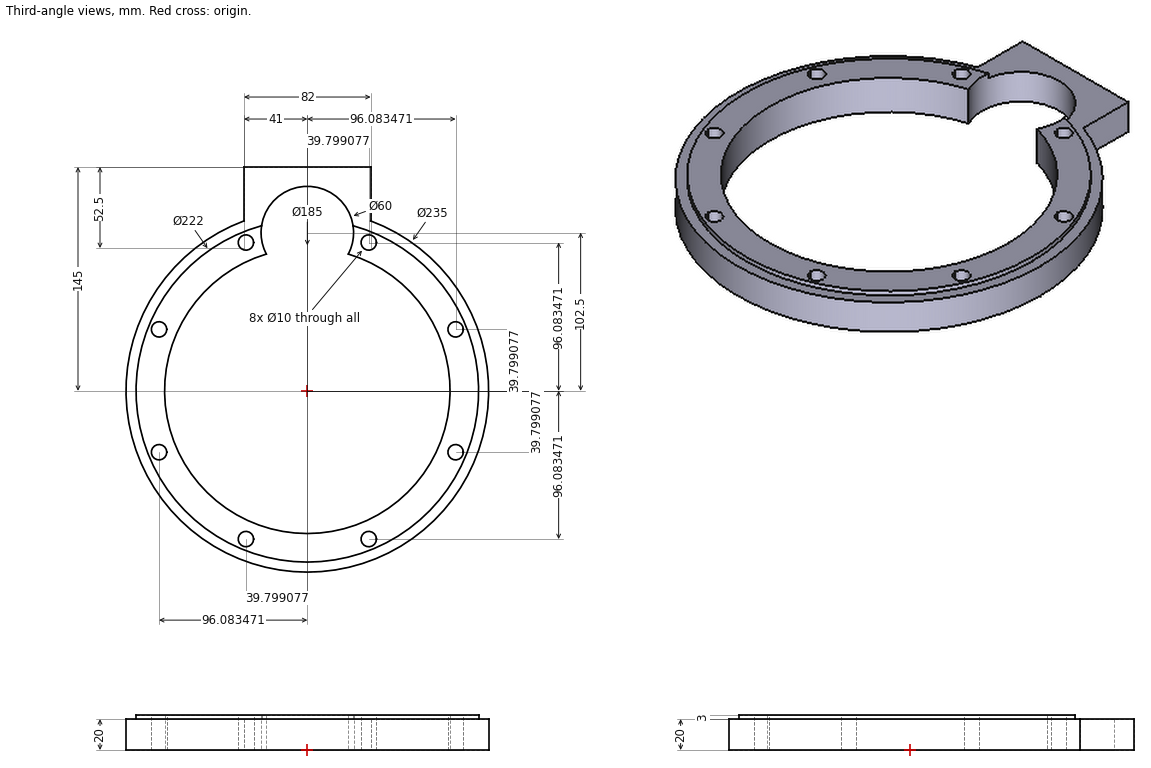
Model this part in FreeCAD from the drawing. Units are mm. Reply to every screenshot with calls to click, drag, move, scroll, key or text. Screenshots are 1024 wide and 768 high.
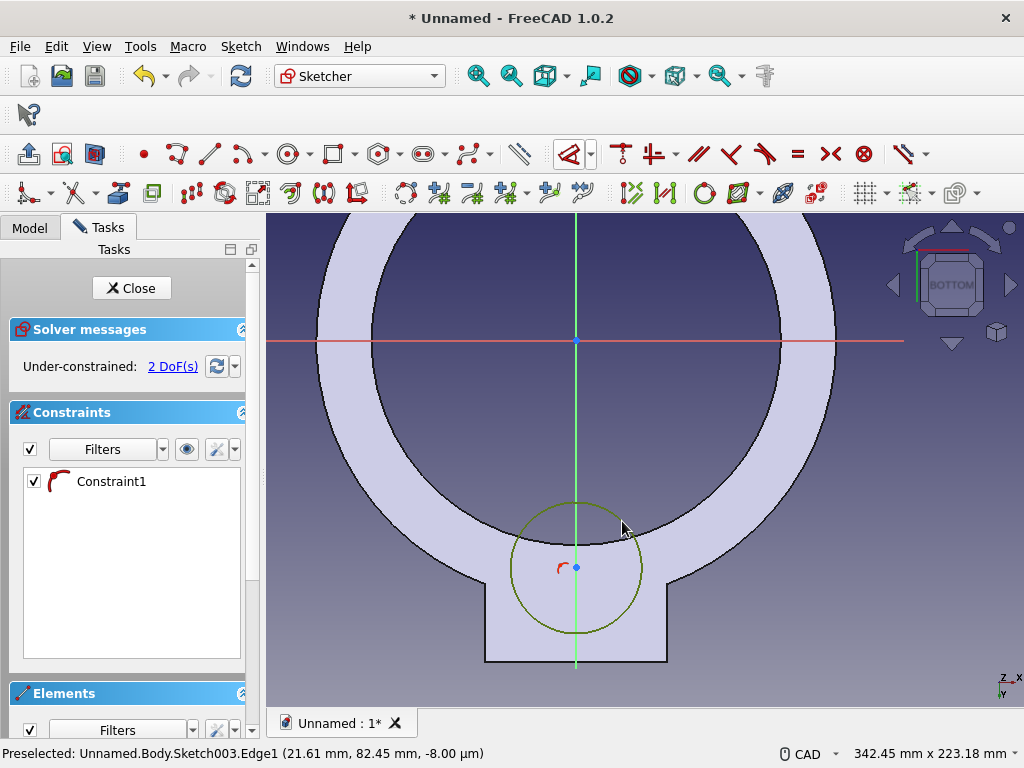
key(k)
key(o)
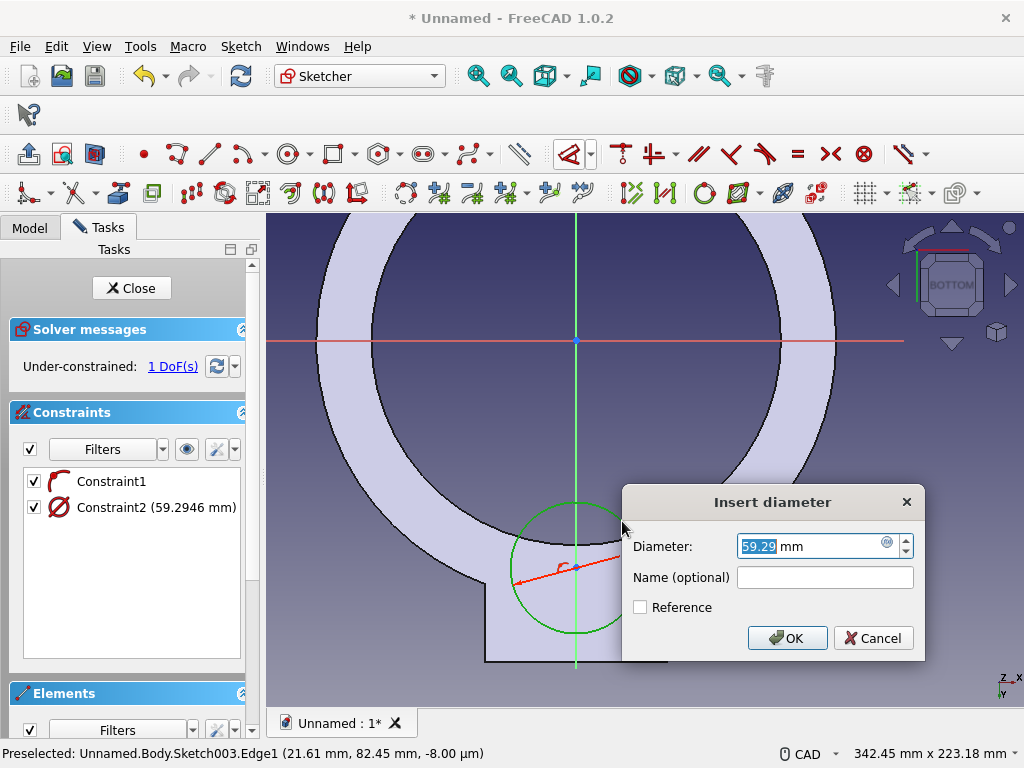
text(60)
key(Return)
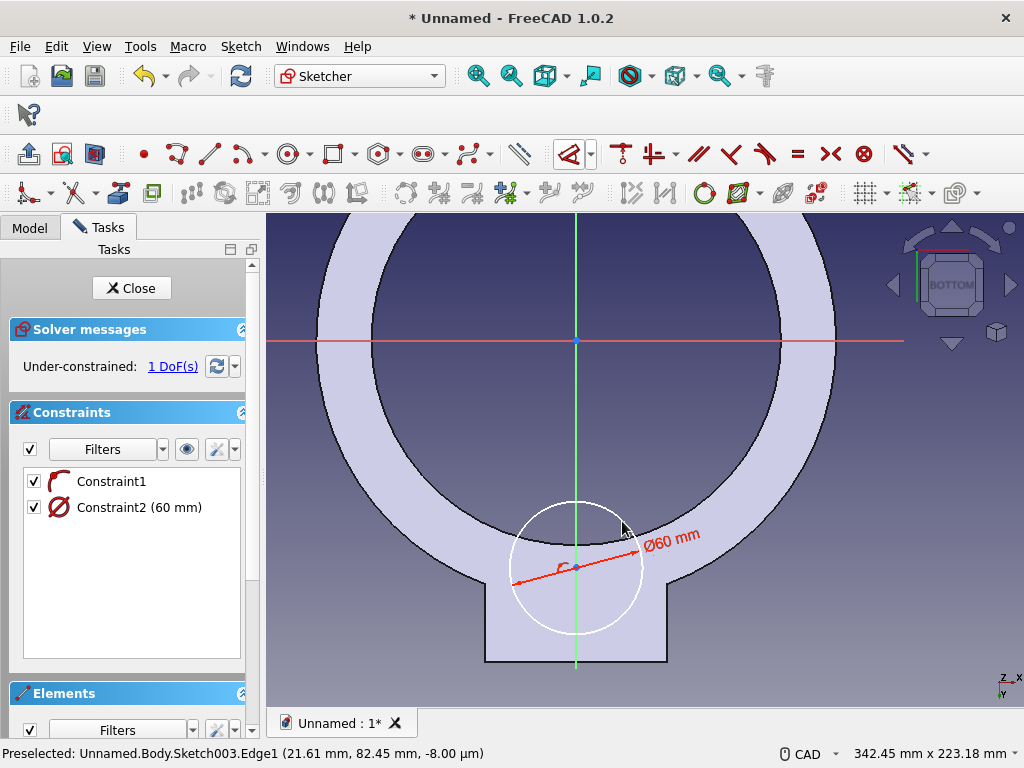
click(576, 568)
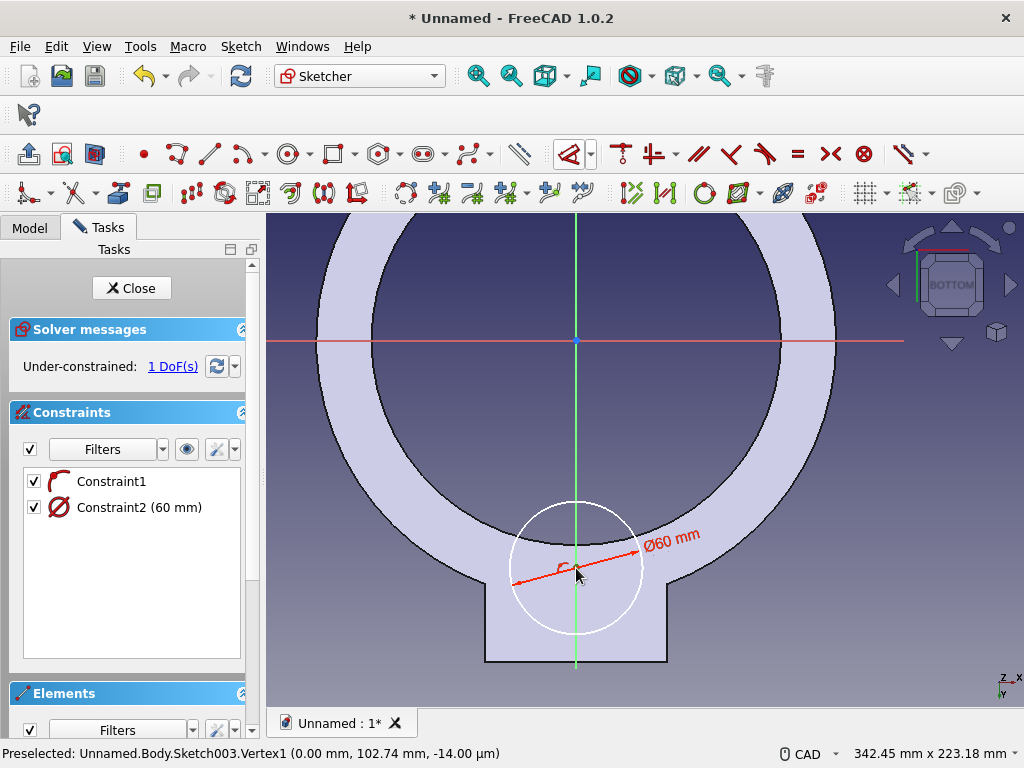
key(i)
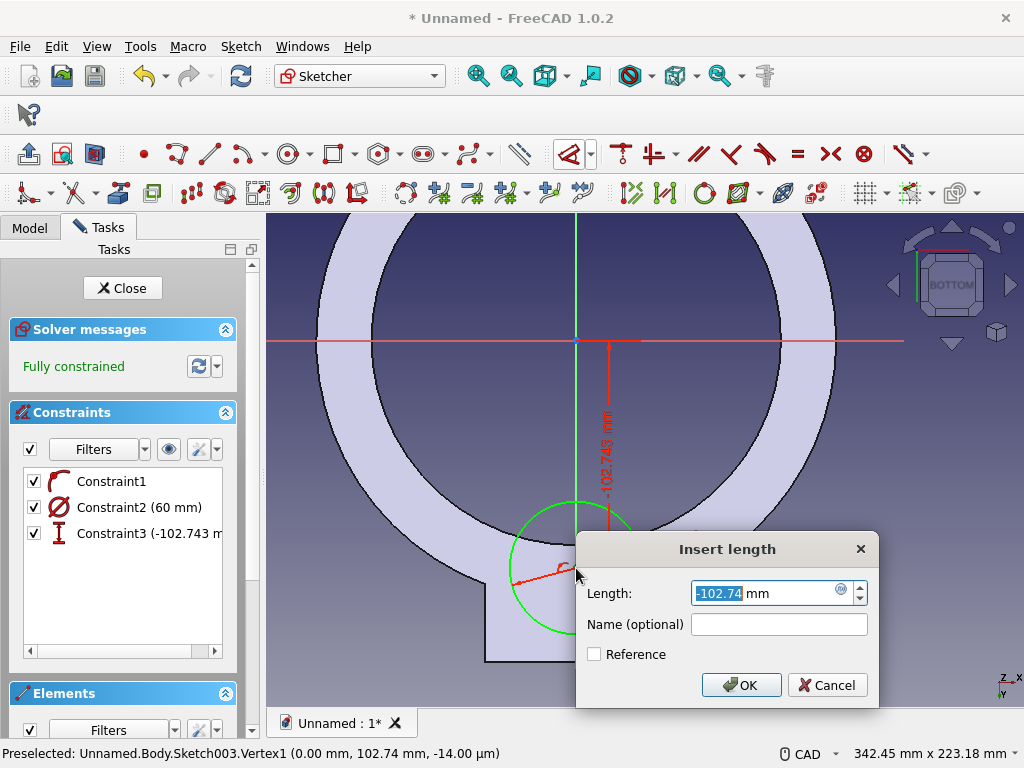
text(-102.5)
key(Return)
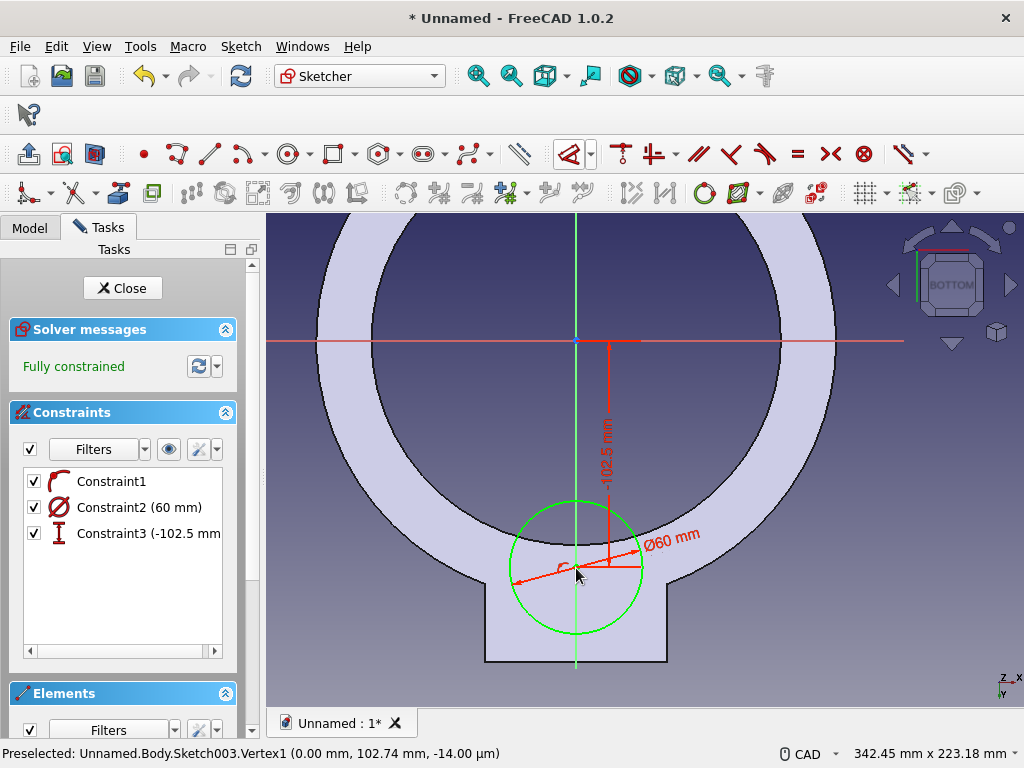
click(123, 288)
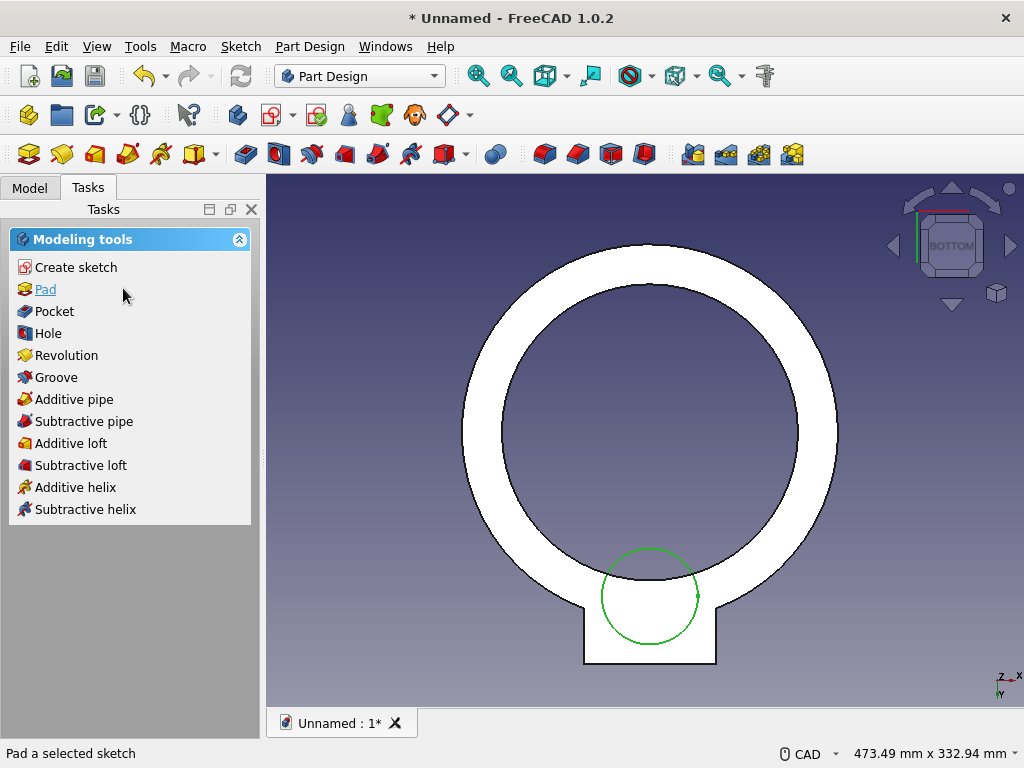
click(246, 154)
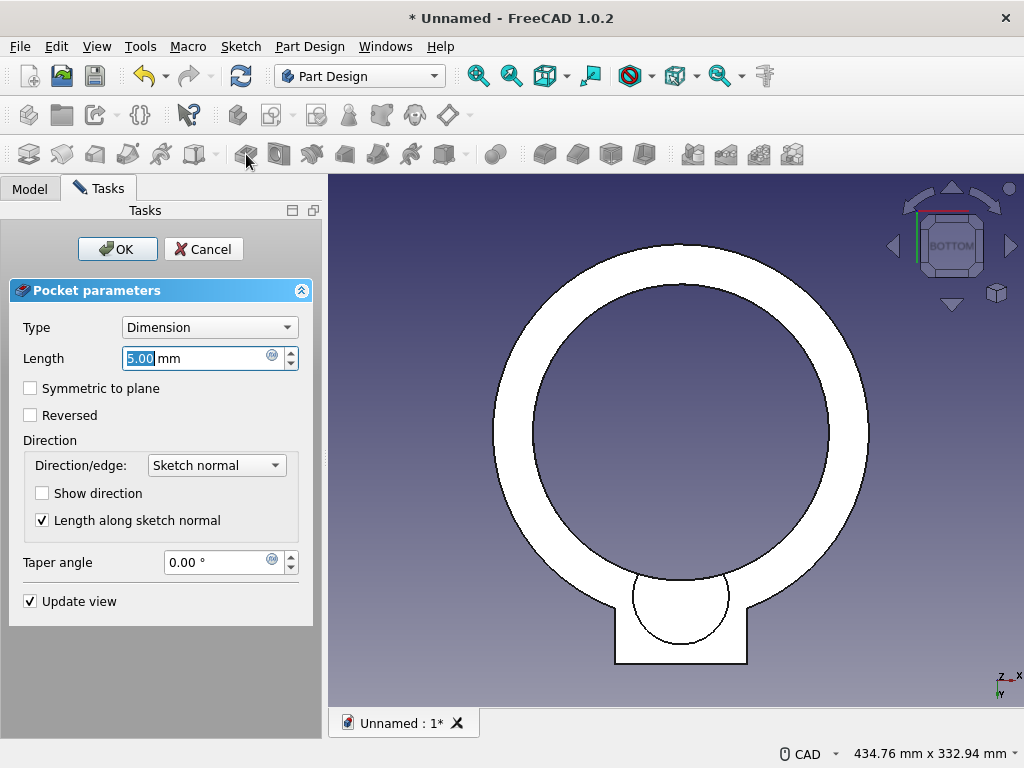
click(210, 328)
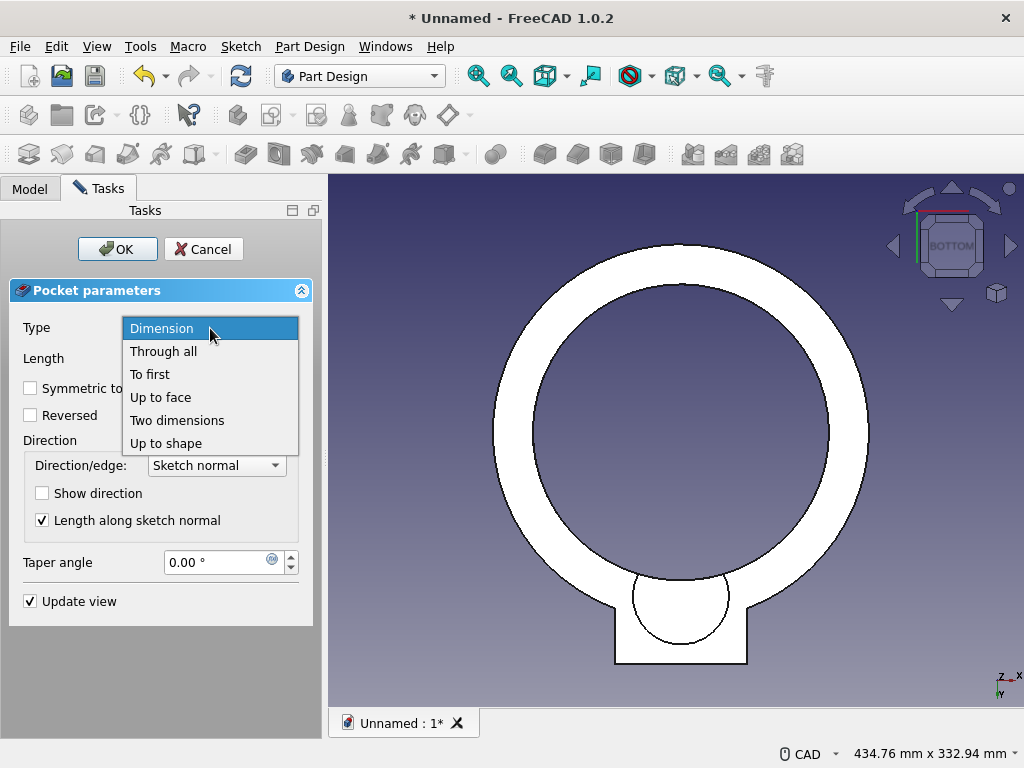
click(208, 352)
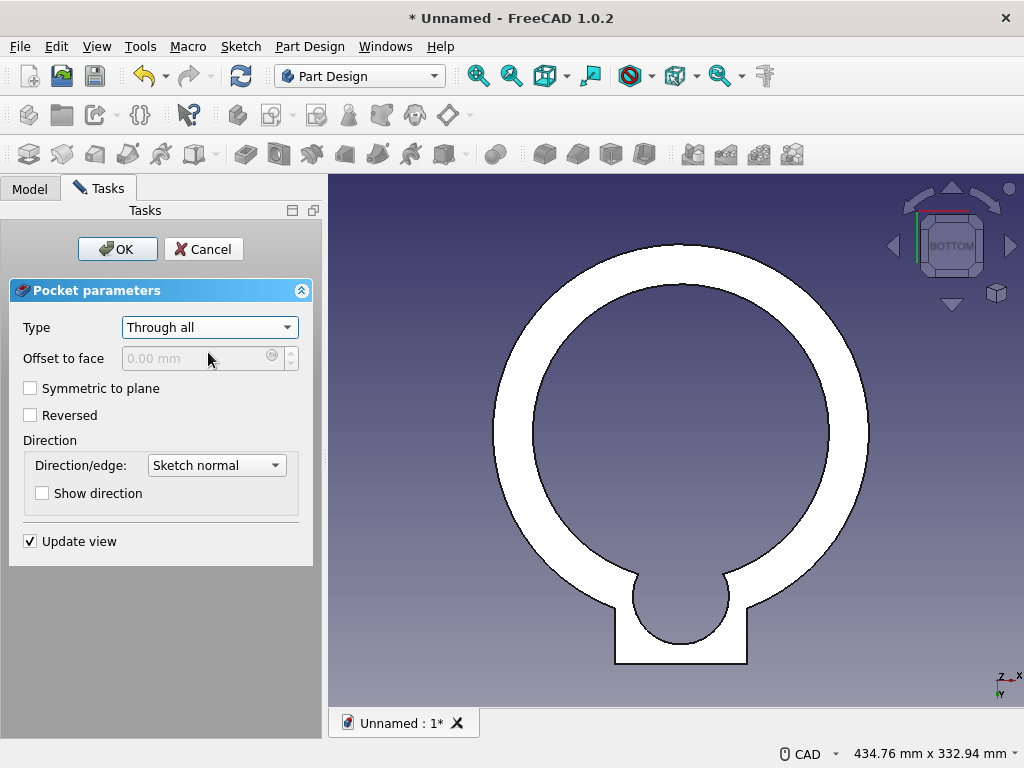
click(118, 249)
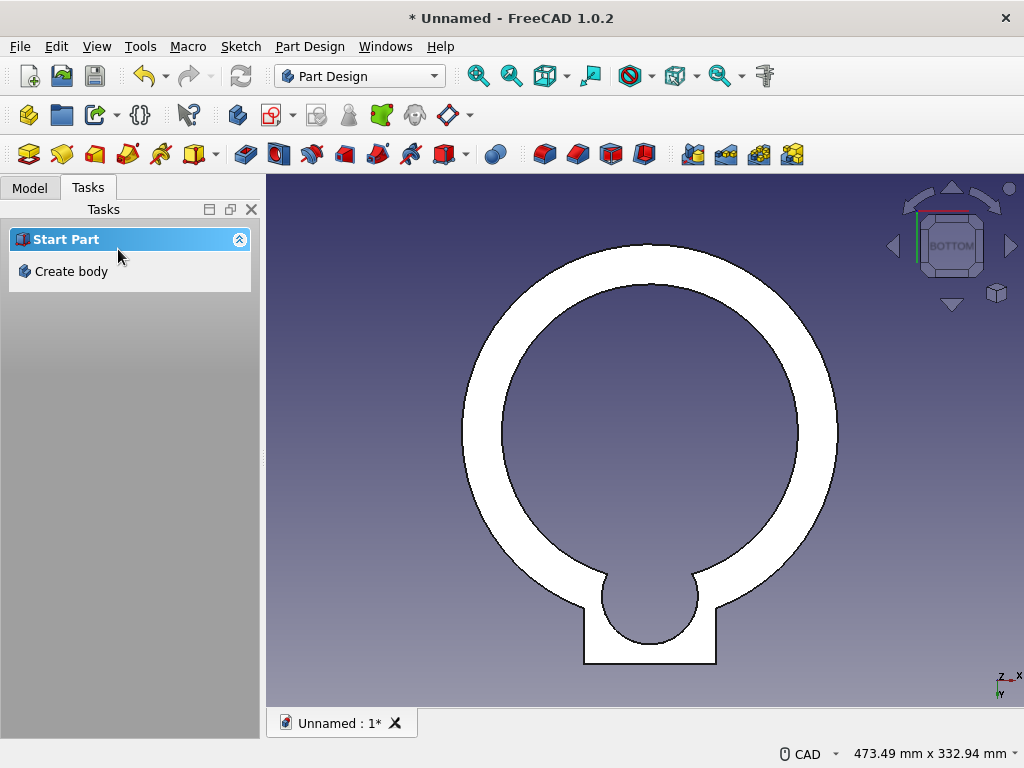
click(704, 273)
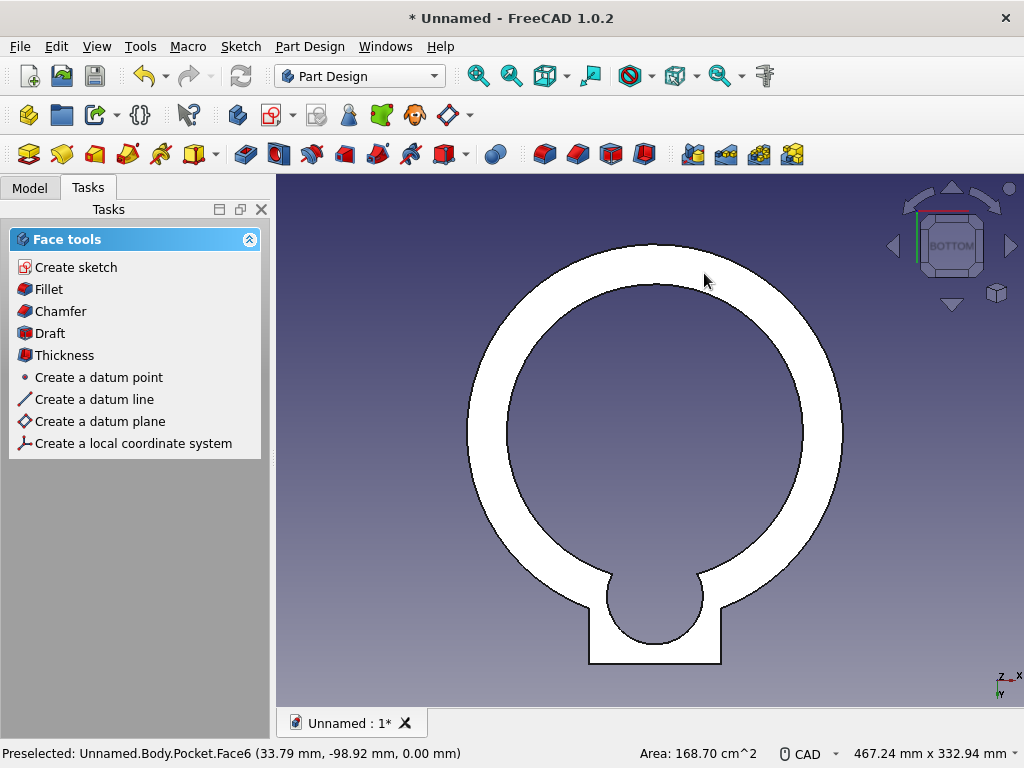
click(270, 116)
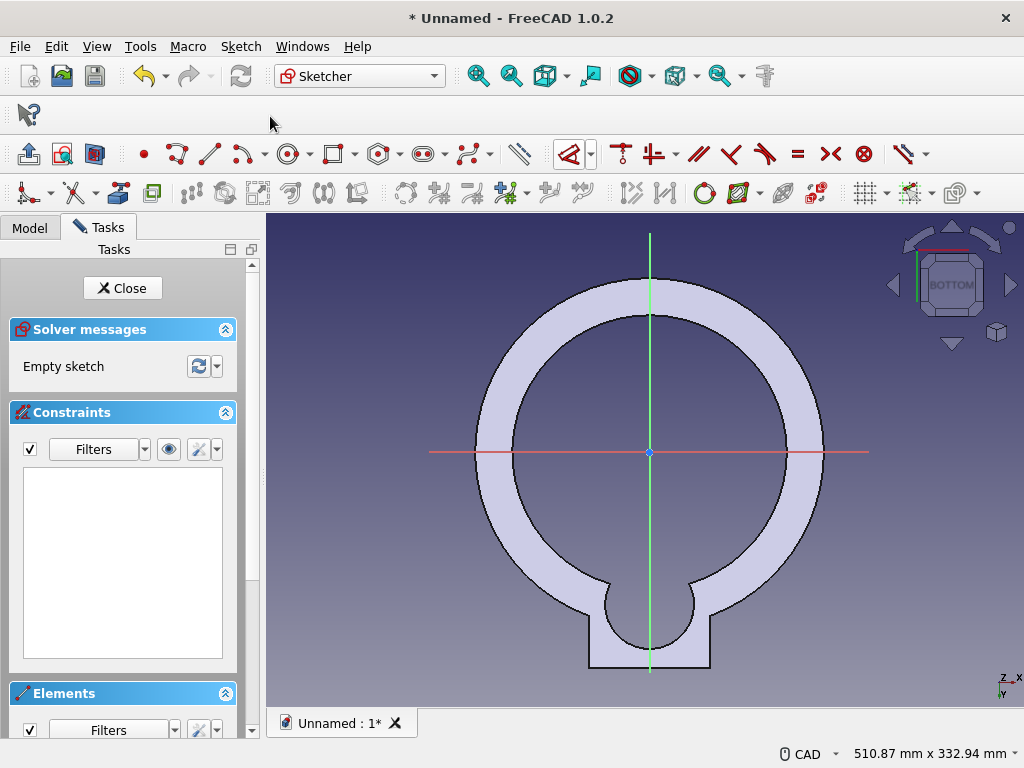
click(288, 154)